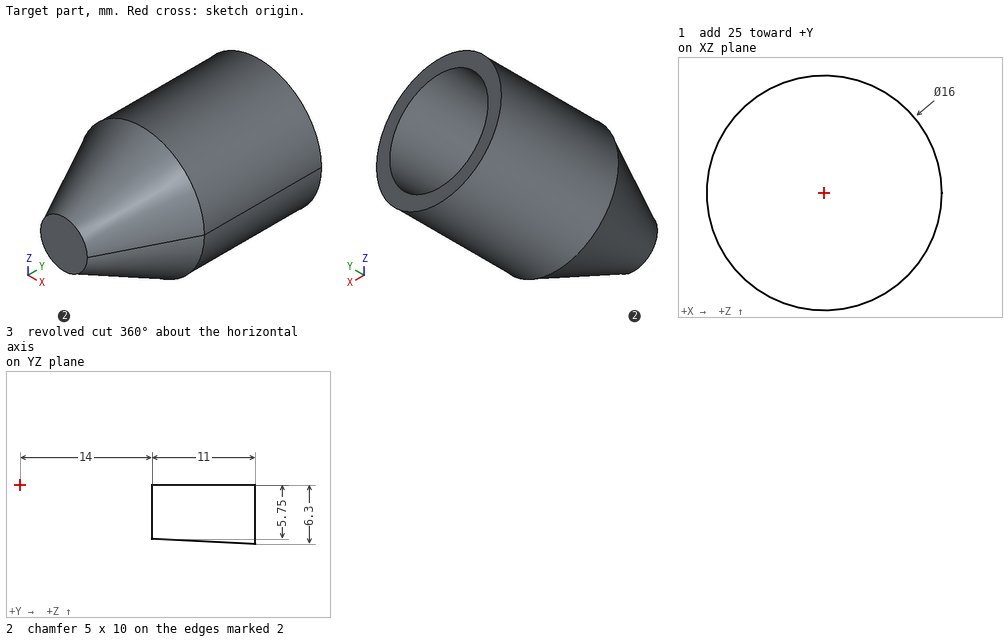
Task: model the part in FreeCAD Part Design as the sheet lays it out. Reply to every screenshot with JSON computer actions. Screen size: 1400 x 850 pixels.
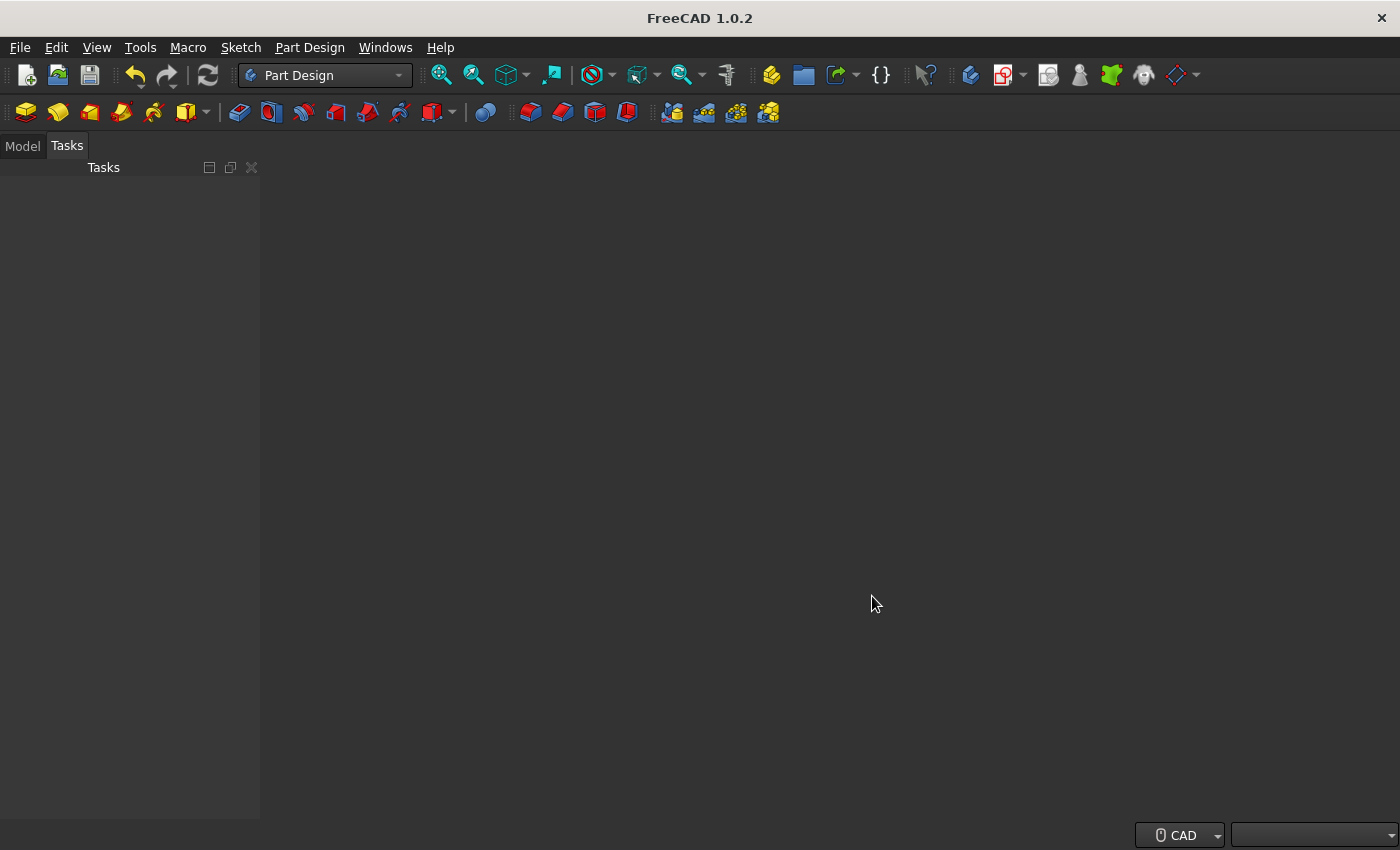
{"action": "left_click", "coordinate": [26, 76]}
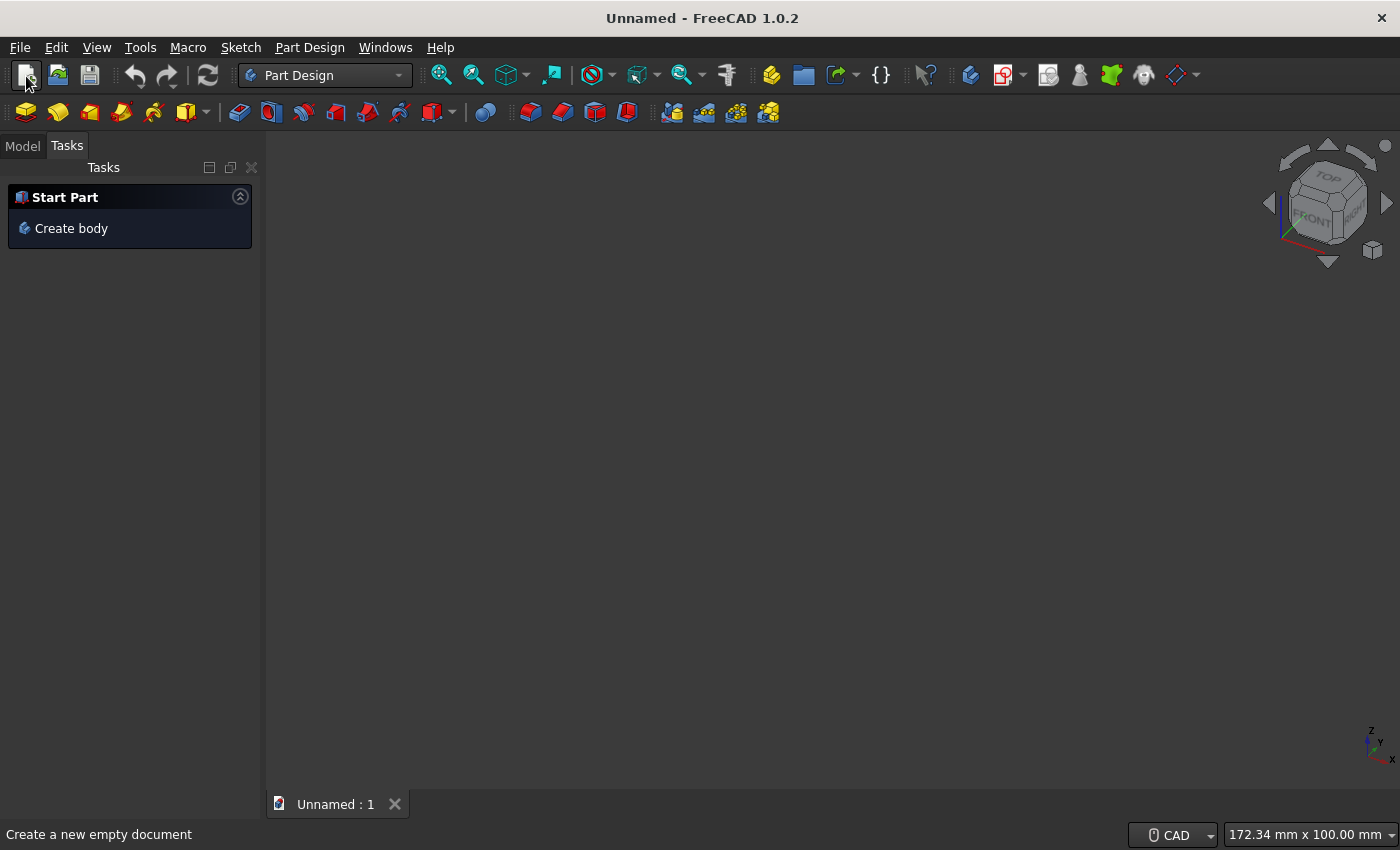
{"action": "left_click", "coordinate": [1004, 76]}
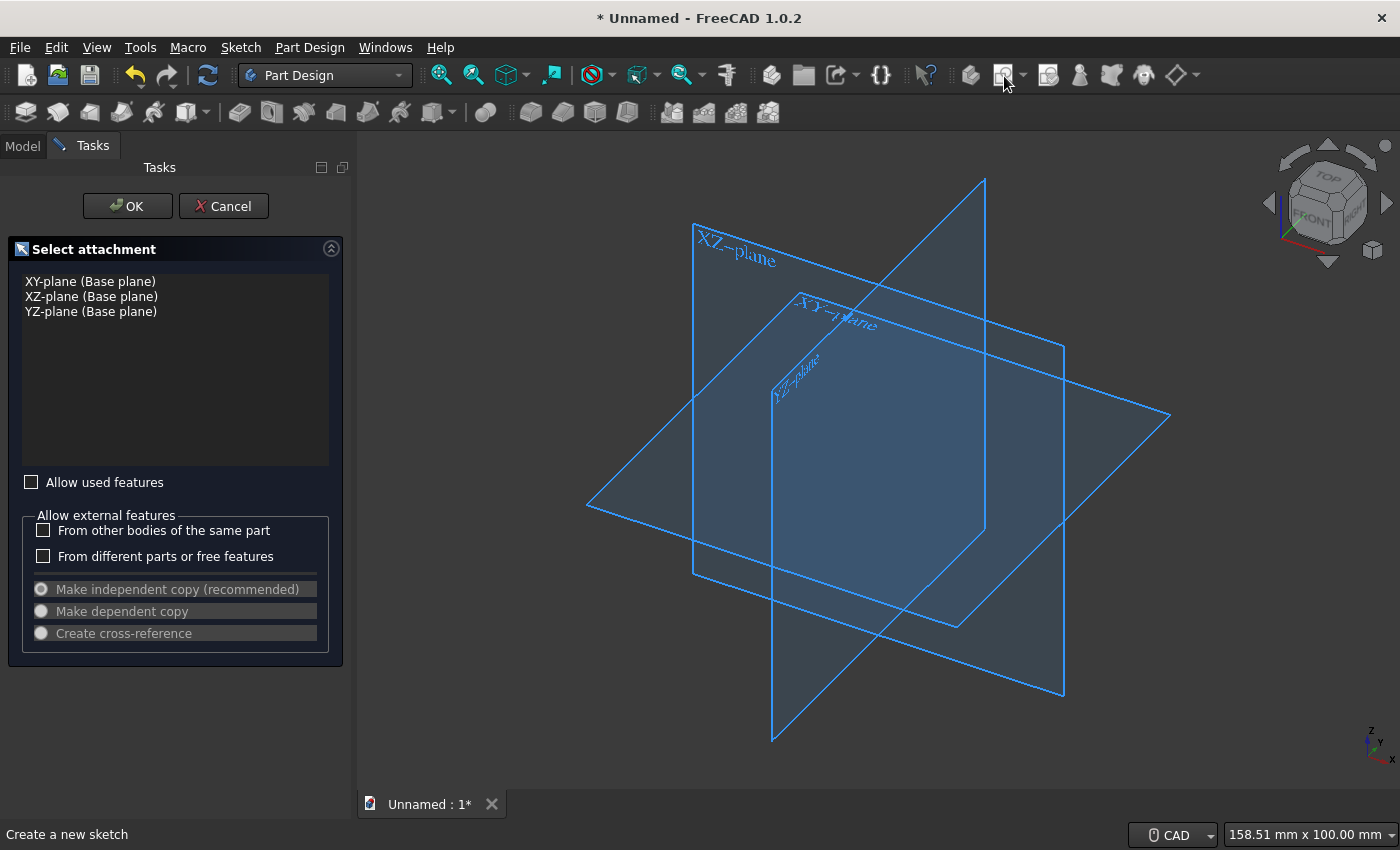
{"action": "left_click", "coordinate": [82, 296]}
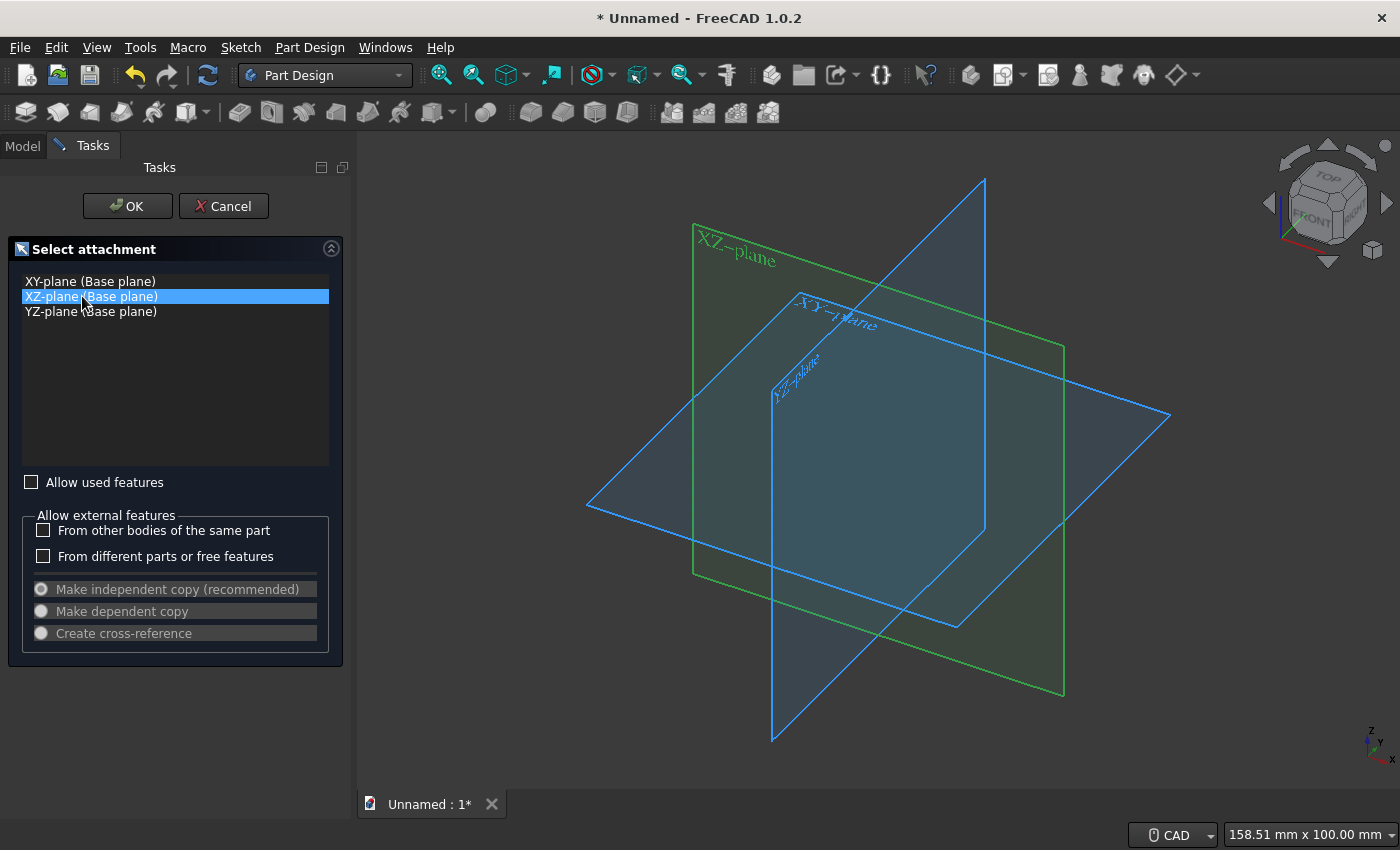
{"action": "left_click", "coordinate": [128, 206]}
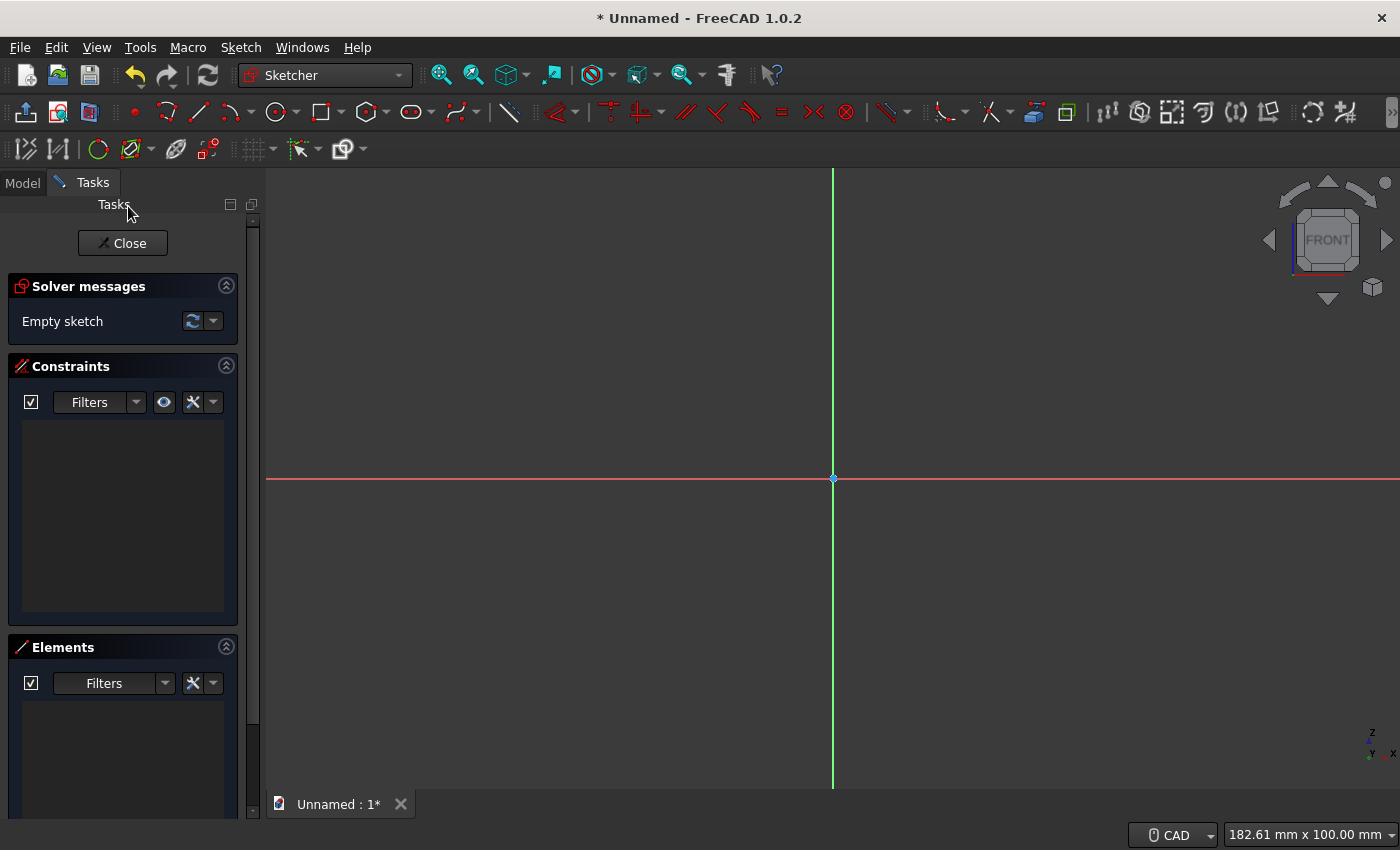
{"action": "scroll", "coordinate": [855, 479], "scroll_direction": "up", "scroll_amount": 7}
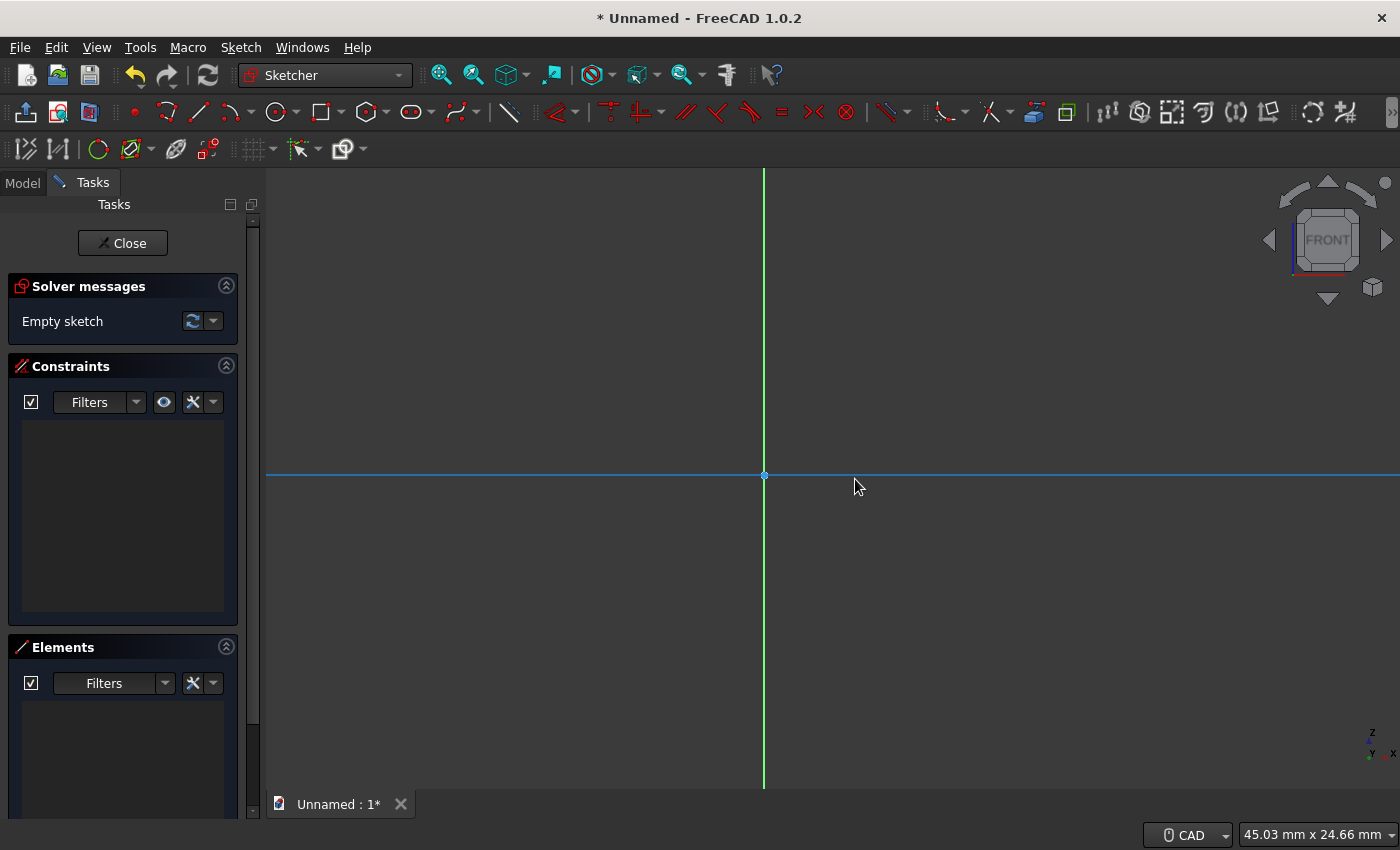
{"action": "left_click", "coordinate": [276, 112]}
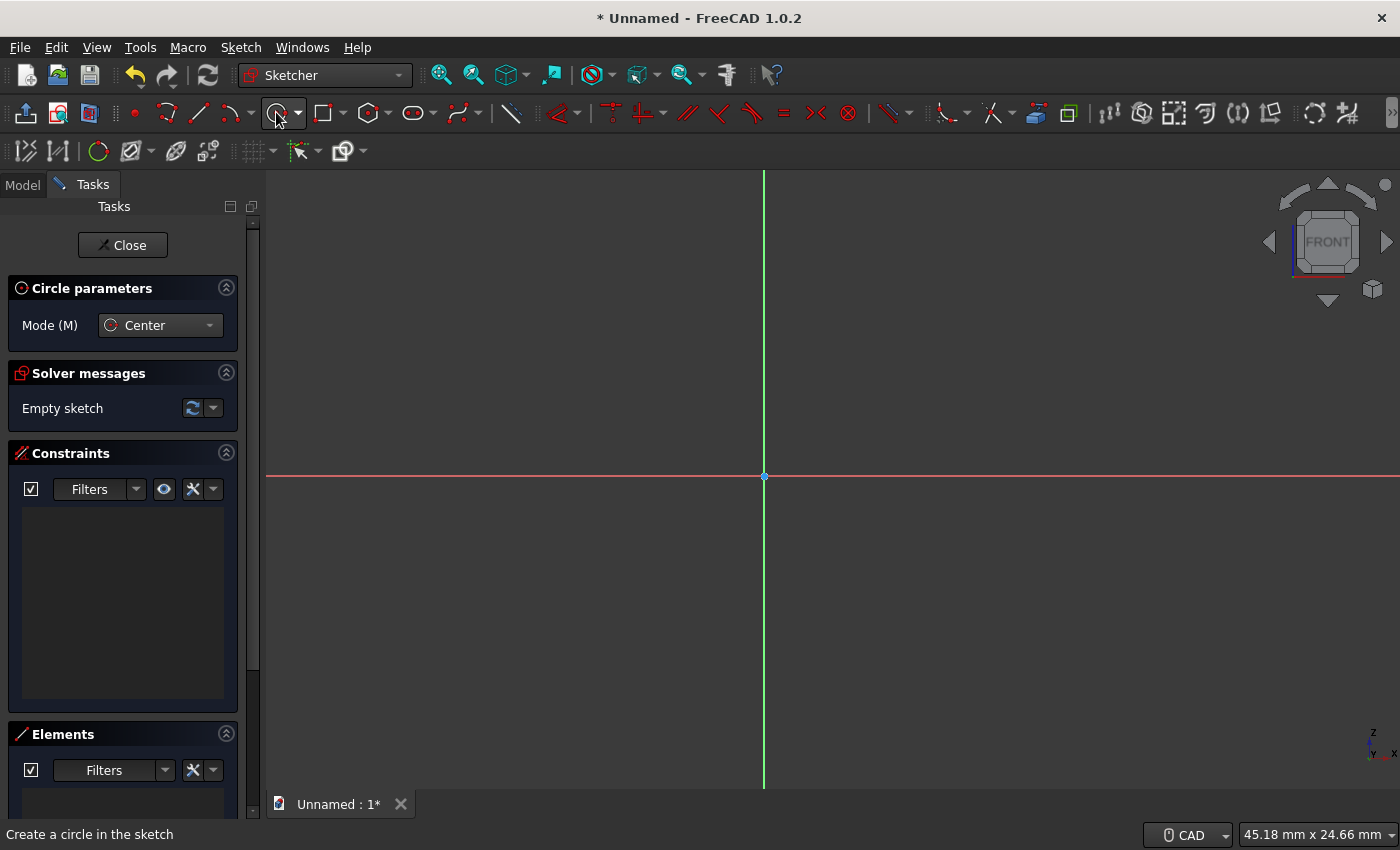
{"action": "left_click", "coordinate": [764, 476]}
{"action": "left_click", "coordinate": [906, 334]}
{"action": "key", "text": "Escape"}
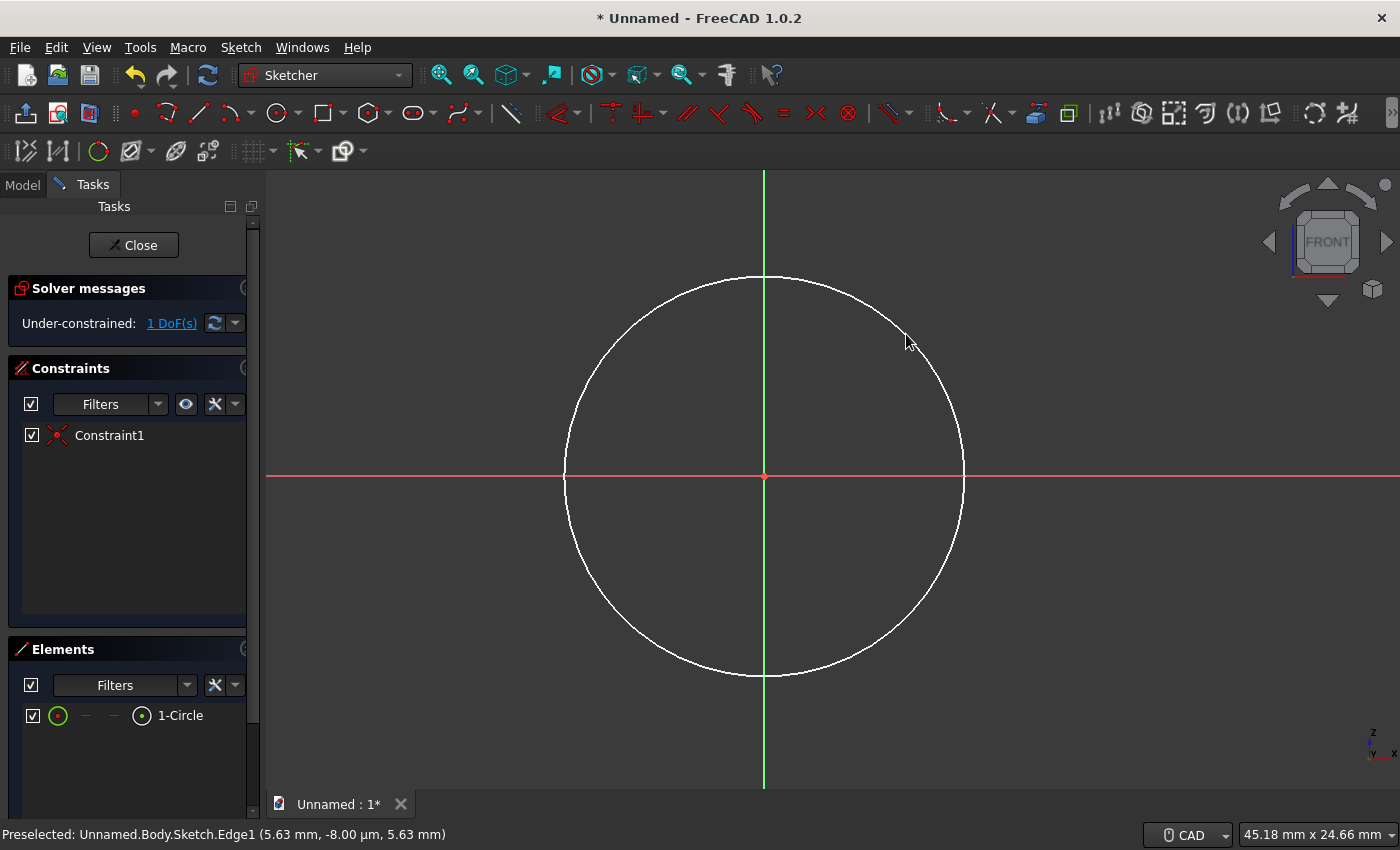
{"action": "left_click", "coordinate": [558, 114]}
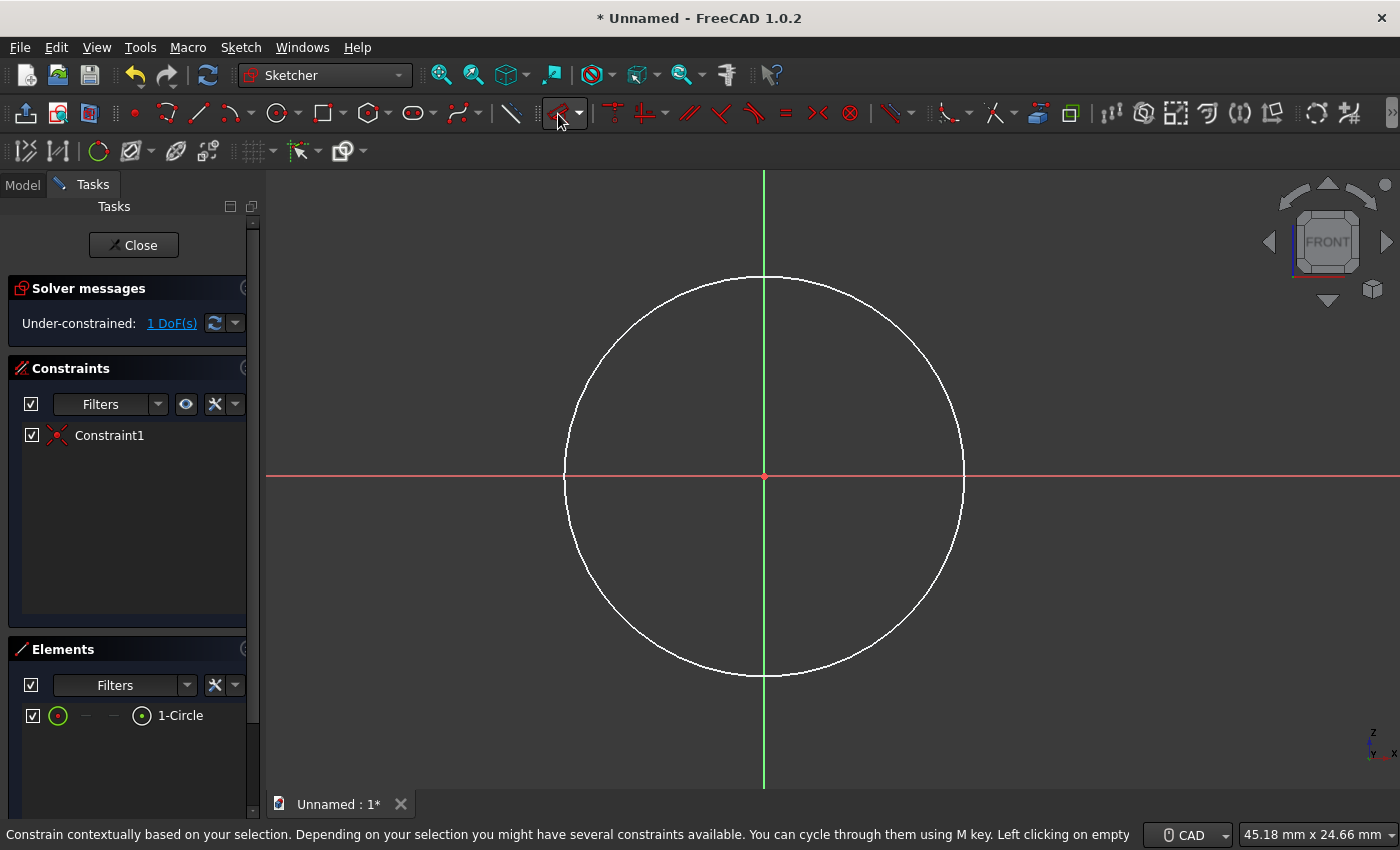
{"action": "left_click", "coordinate": [905, 334]}
{"action": "left_click", "coordinate": [927, 311]}